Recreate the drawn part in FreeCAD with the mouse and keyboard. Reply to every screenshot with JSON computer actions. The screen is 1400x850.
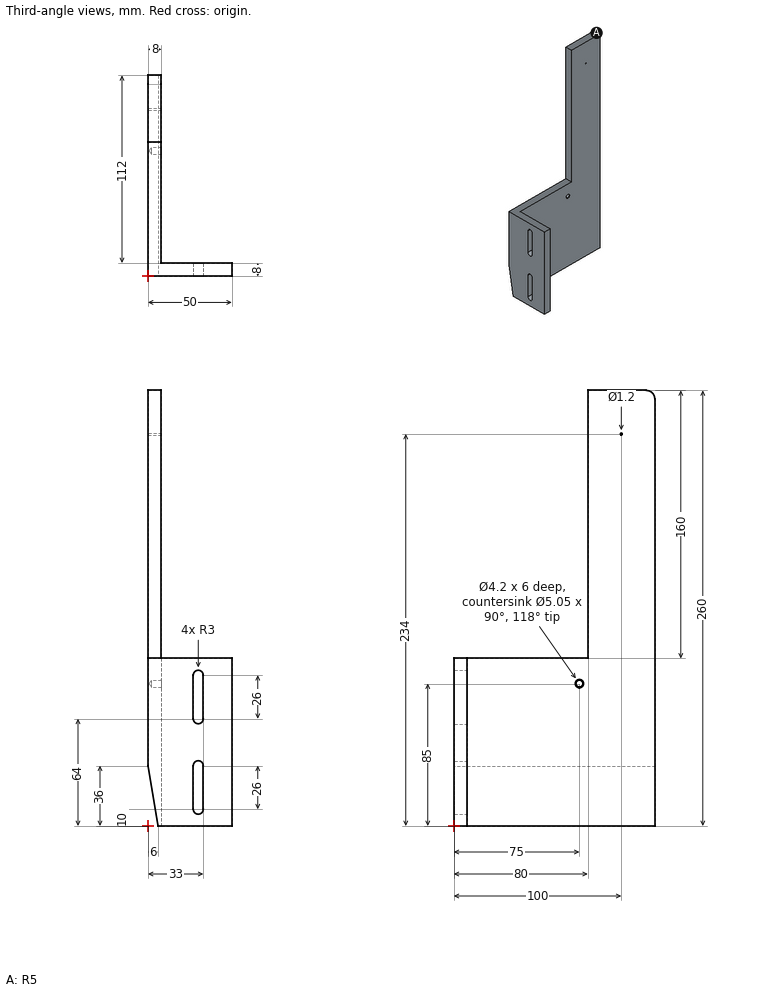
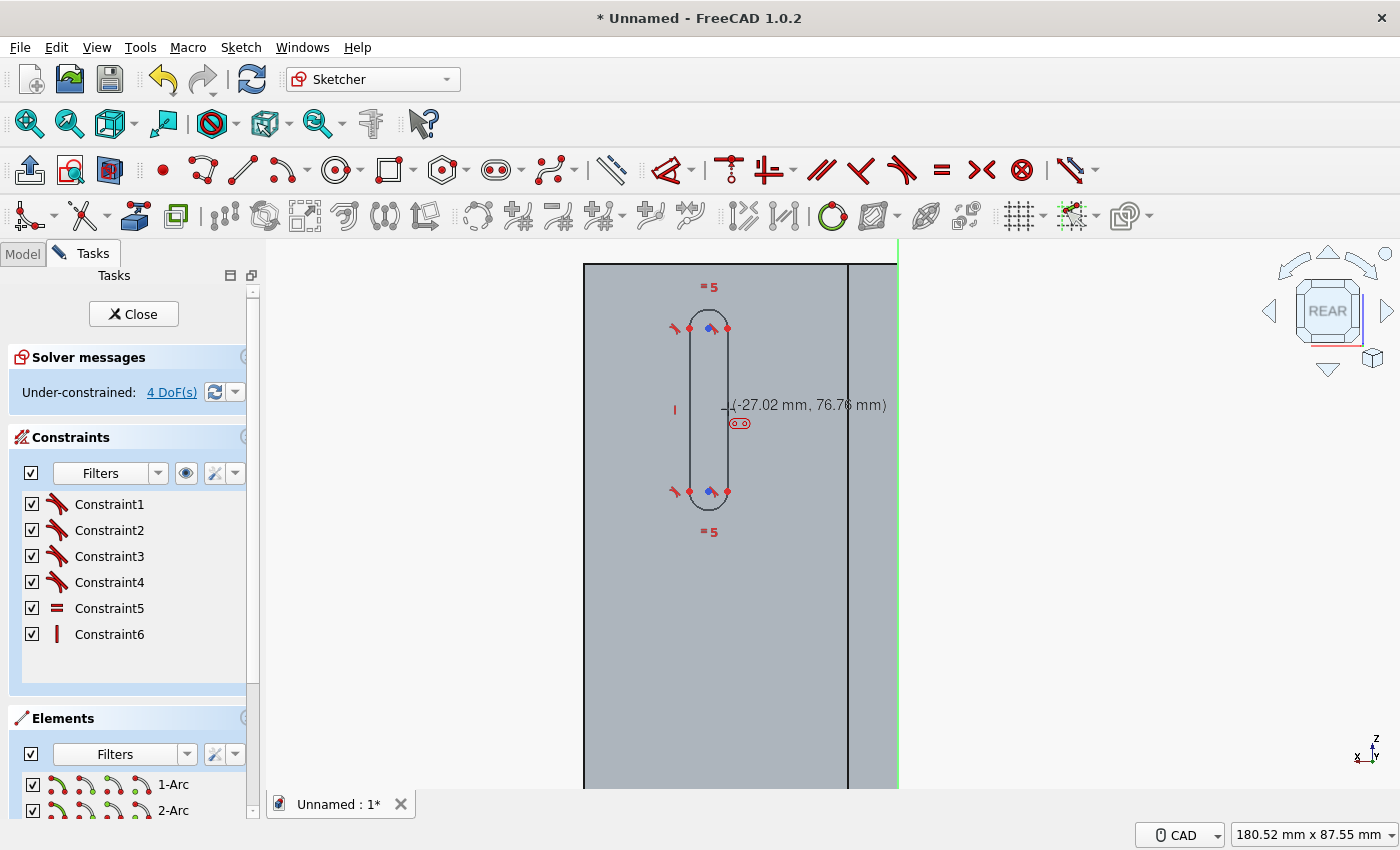
{"action": "scroll", "coordinate": [728, 409], "scroll_direction": "down", "scroll_amount": 3}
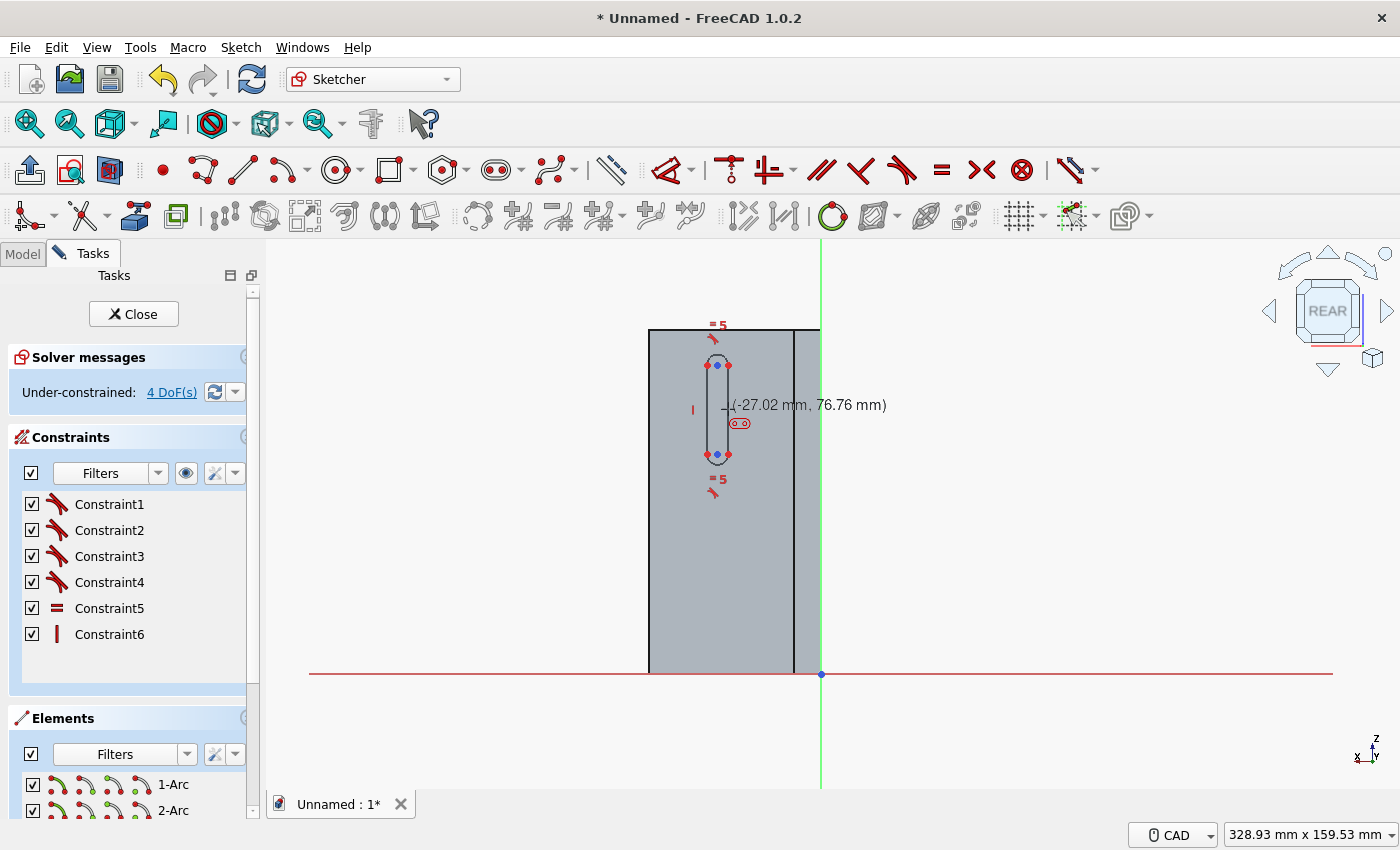
{"action": "scroll", "coordinate": [718, 640], "scroll_direction": "up", "scroll_amount": 4}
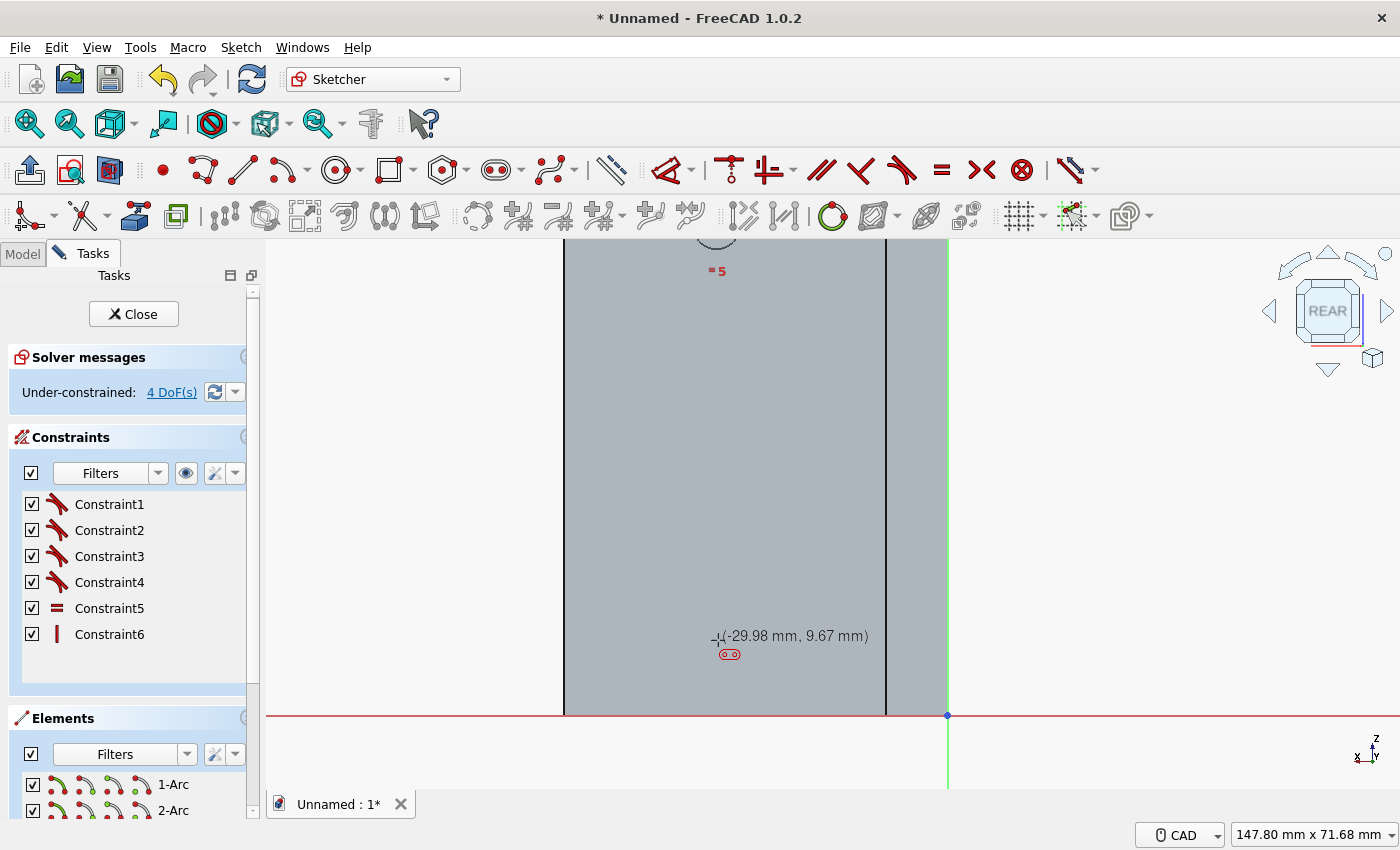
{"action": "left_click", "coordinate": [717, 639]}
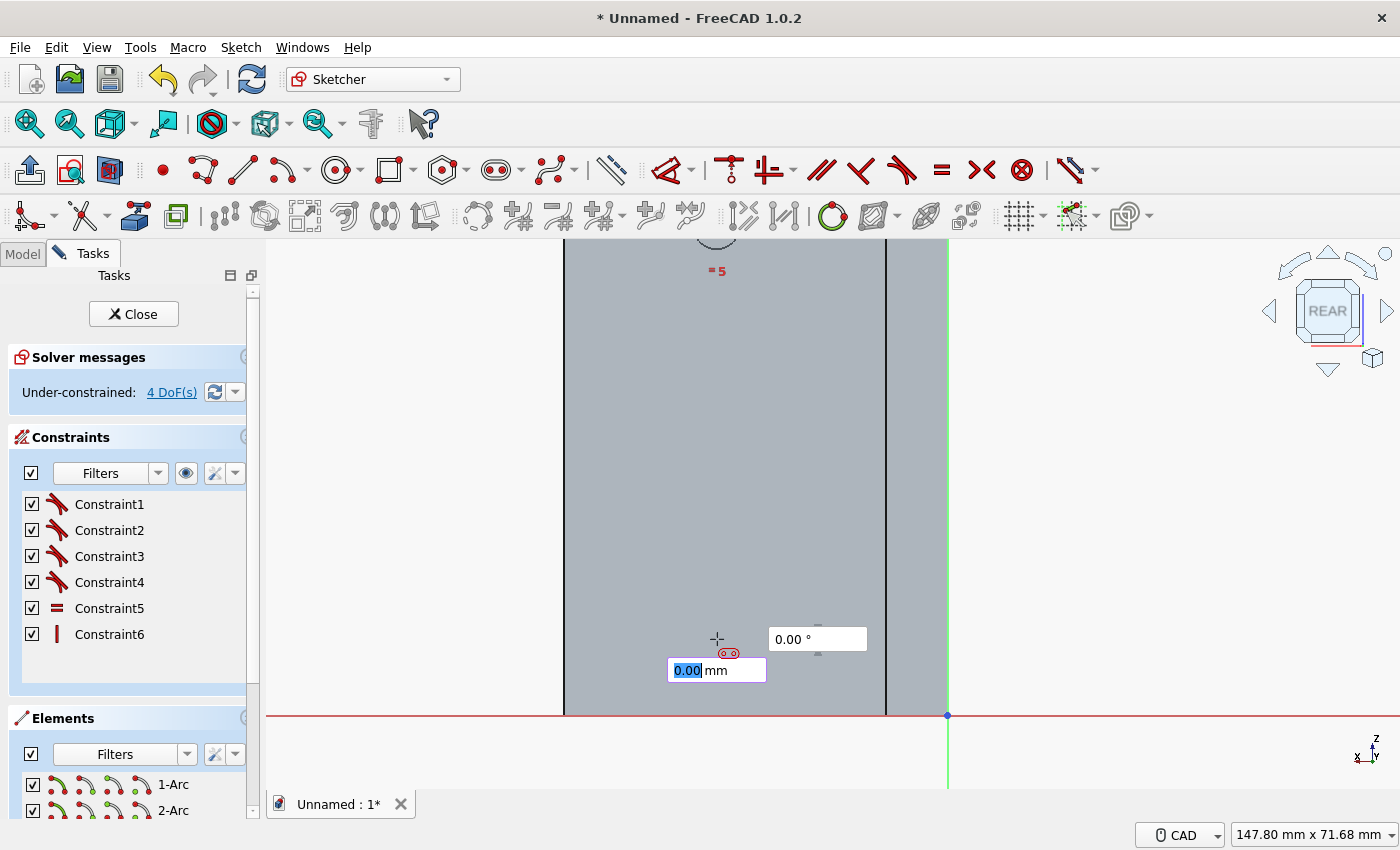
{"action": "left_click", "coordinate": [717, 439]}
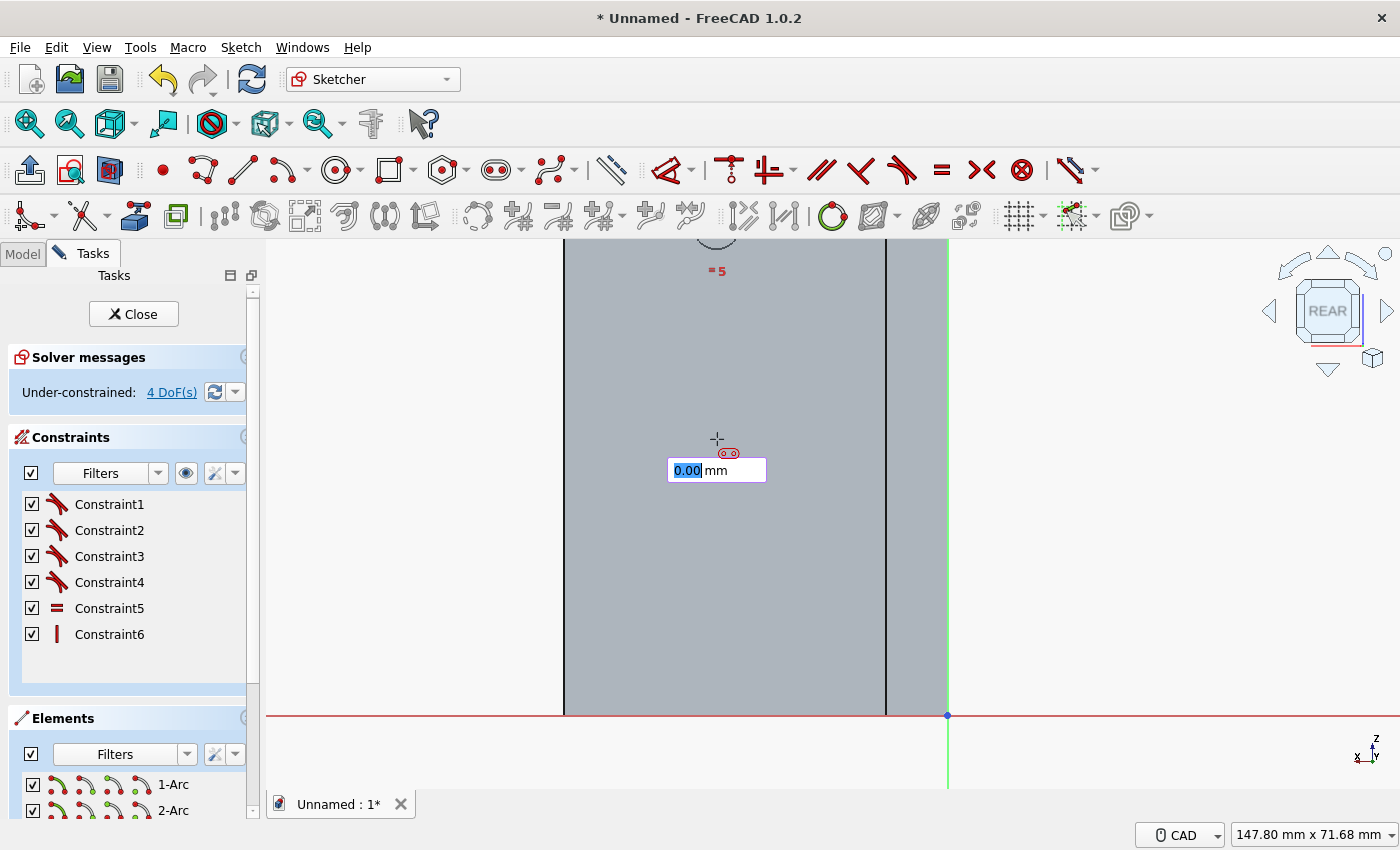
{"action": "left_click", "coordinate": [740, 539]}
{"action": "key", "text": "Escape"}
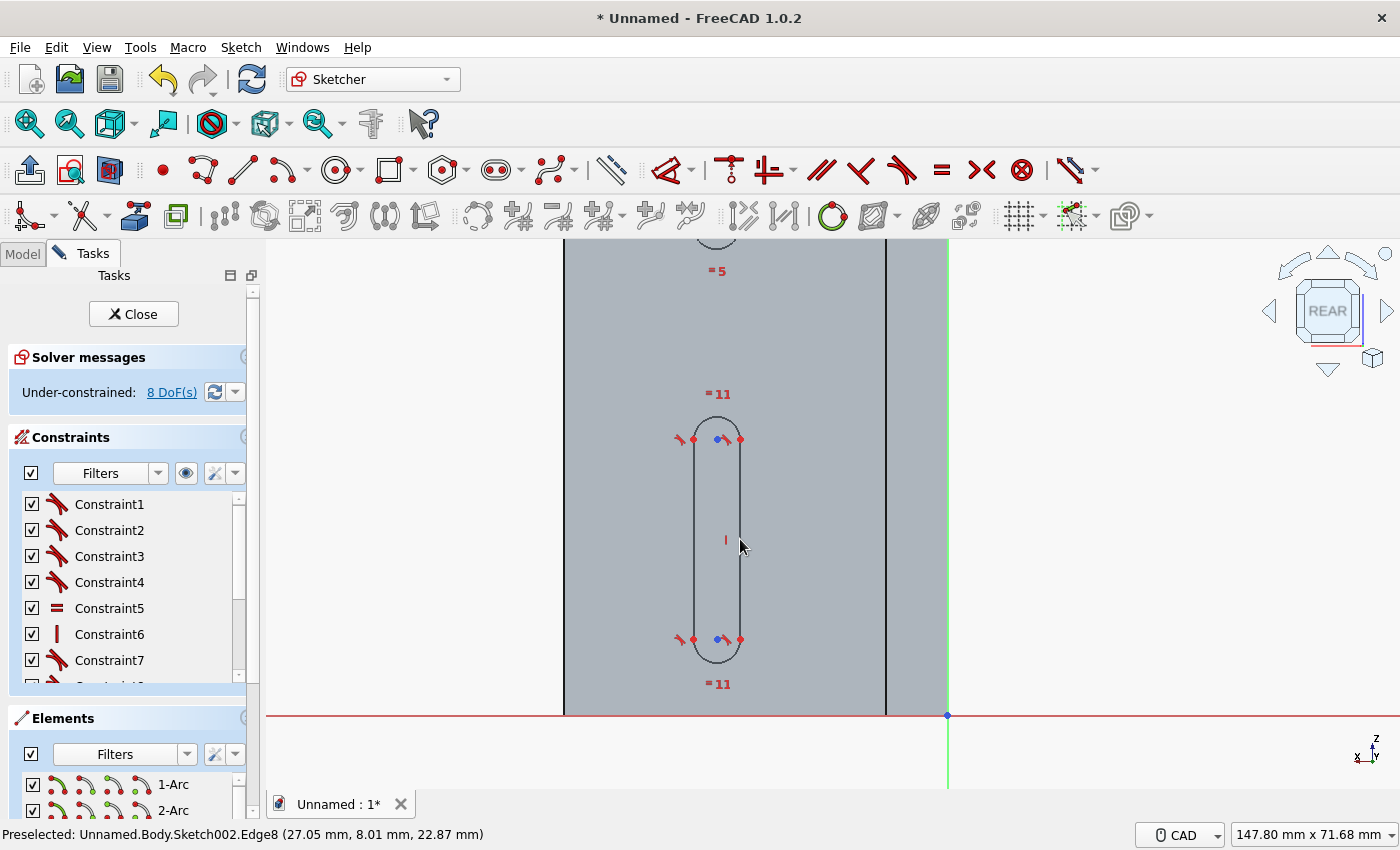
{"action": "scroll", "coordinate": [718, 641], "scroll_direction": "down", "scroll_amount": 4}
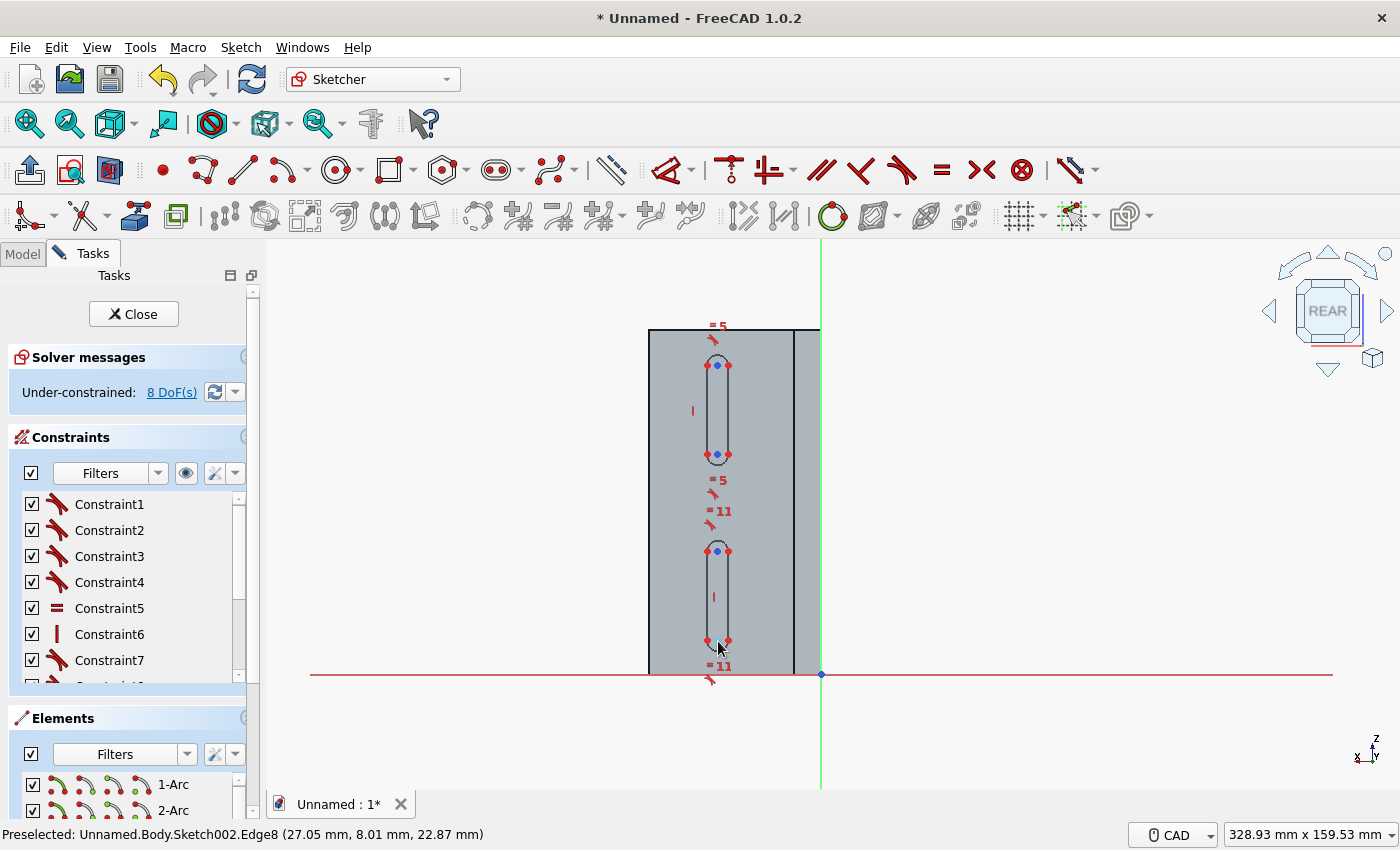
{"action": "scroll", "coordinate": [711, 463], "scroll_direction": "up", "scroll_amount": 2}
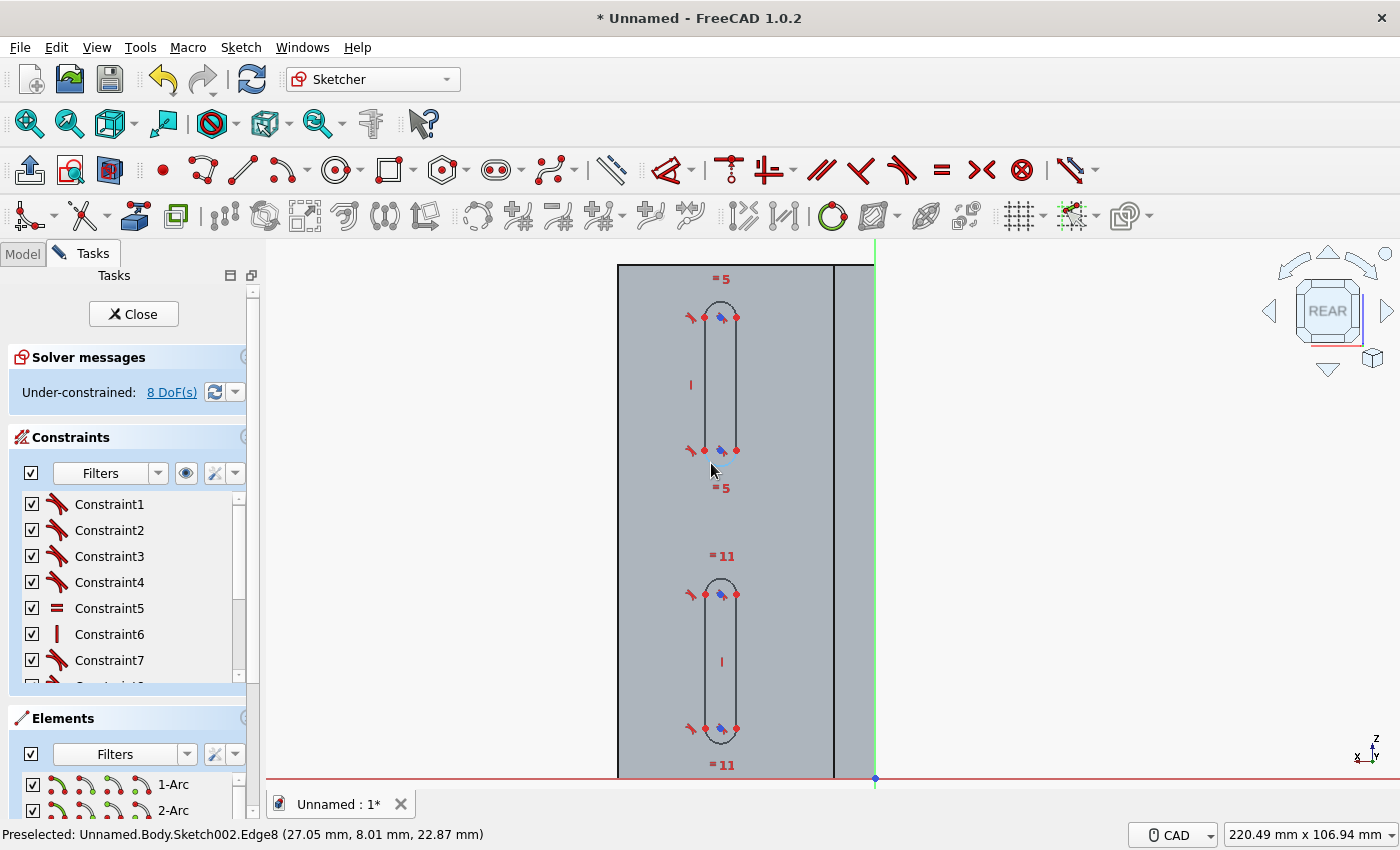
{"action": "left_click", "coordinate": [711, 463]}